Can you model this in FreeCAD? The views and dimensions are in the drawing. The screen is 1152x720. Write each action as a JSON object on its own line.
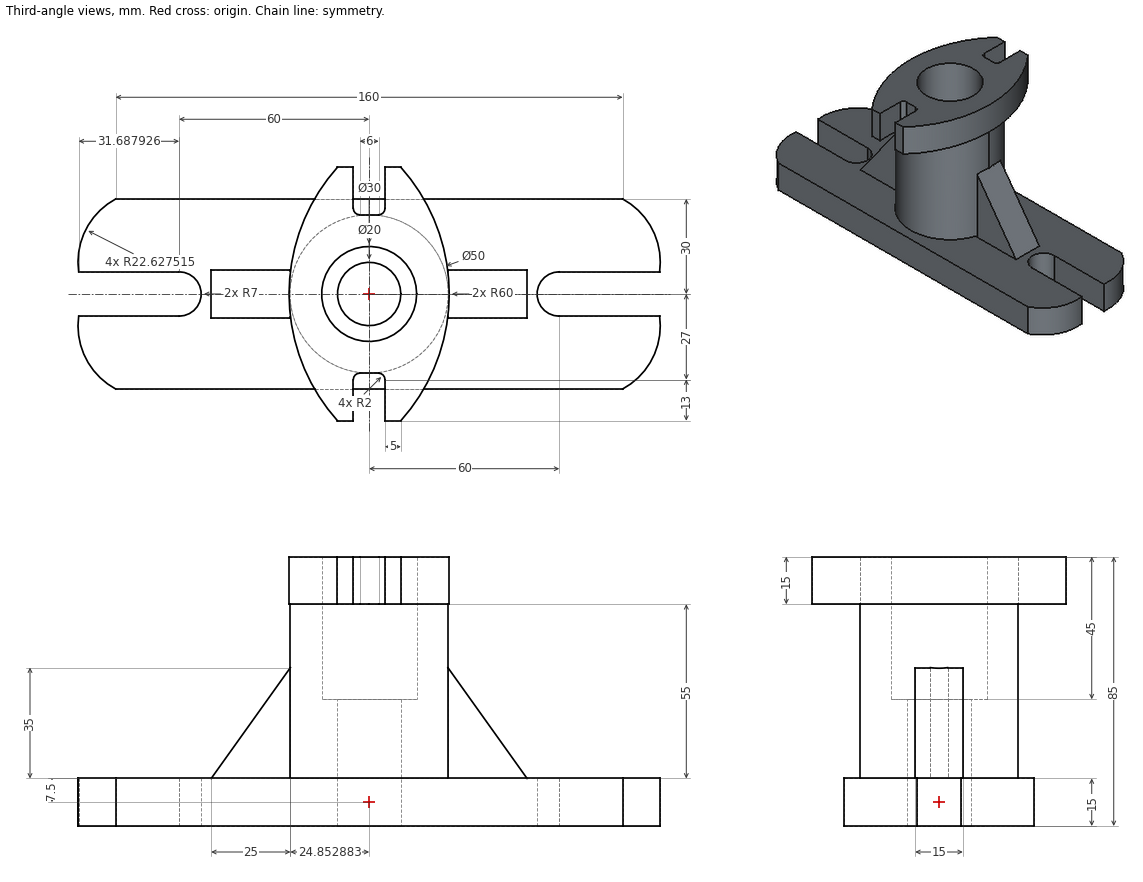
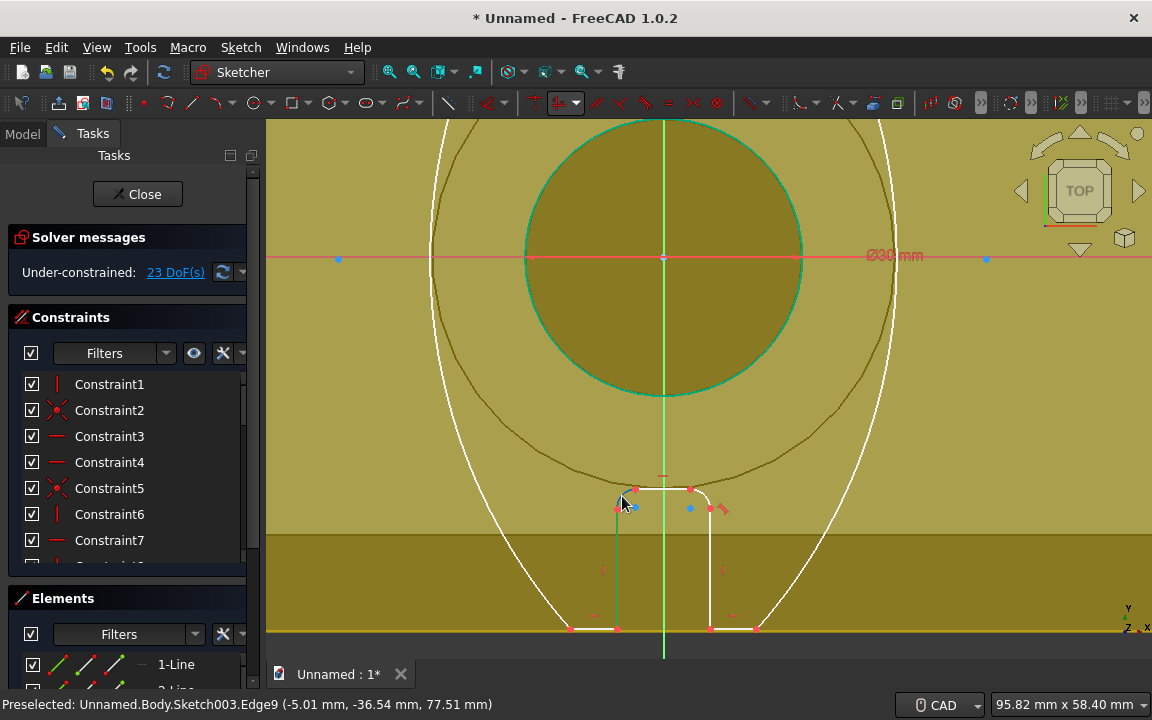
{"action": "left_click", "coordinate": [622, 495]}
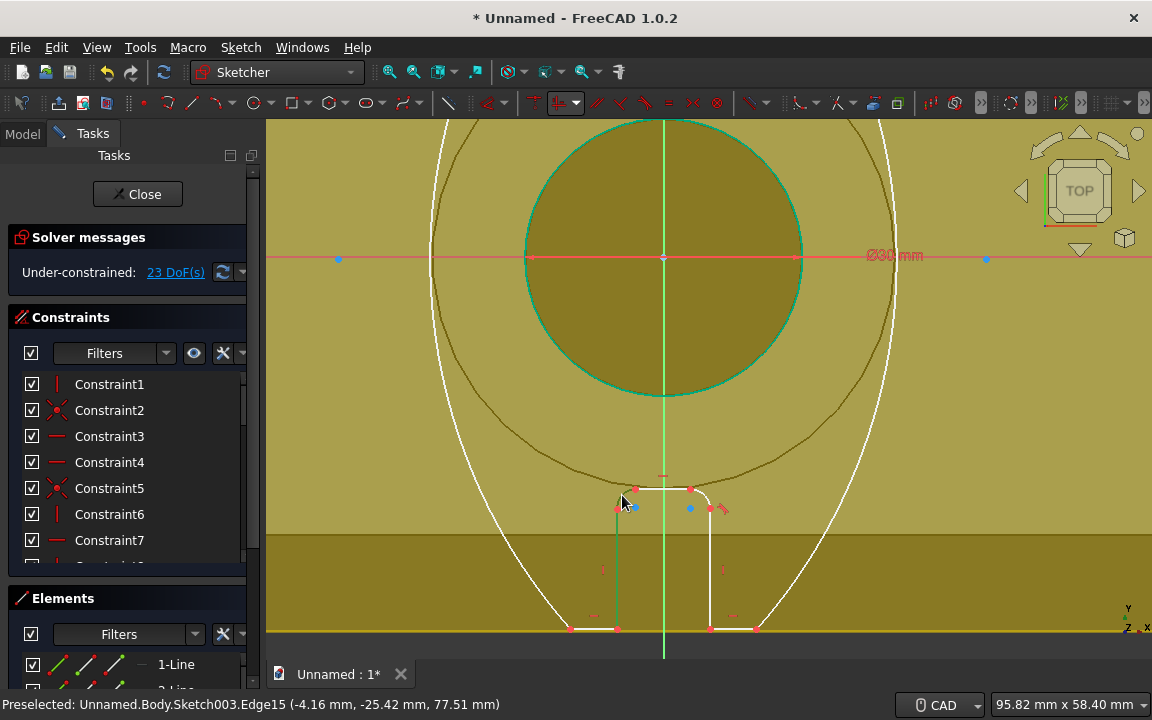
{"action": "key", "text": "t"}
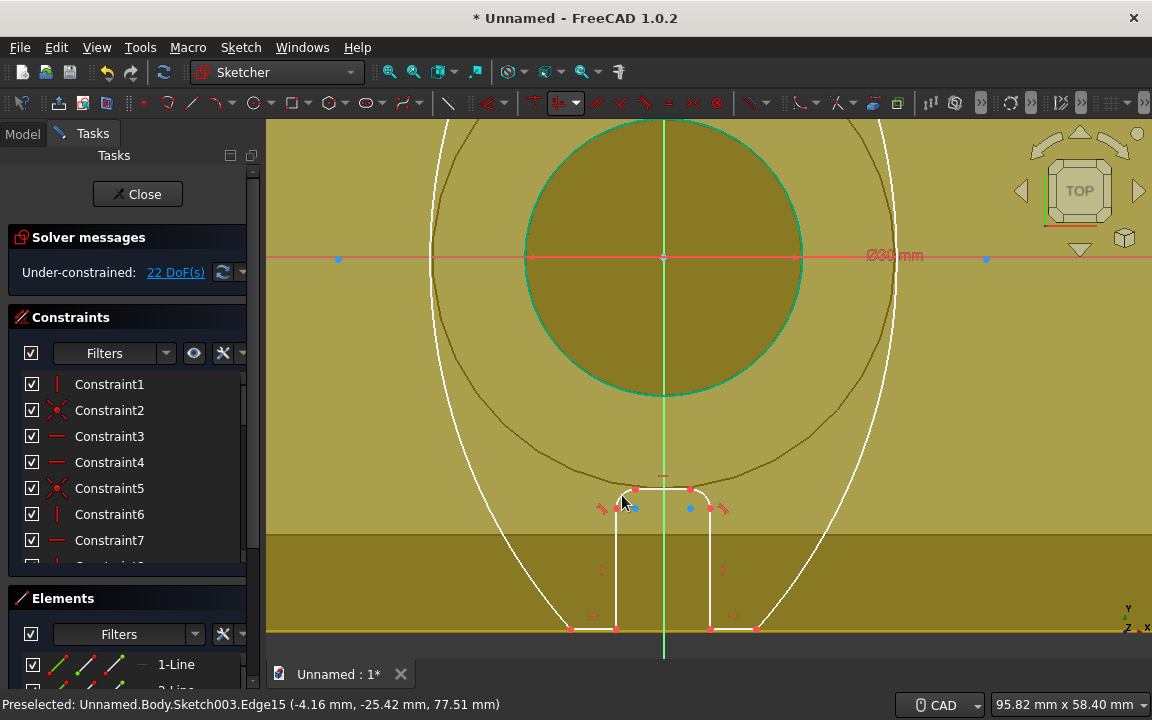
{"action": "left_click", "coordinate": [652, 489]}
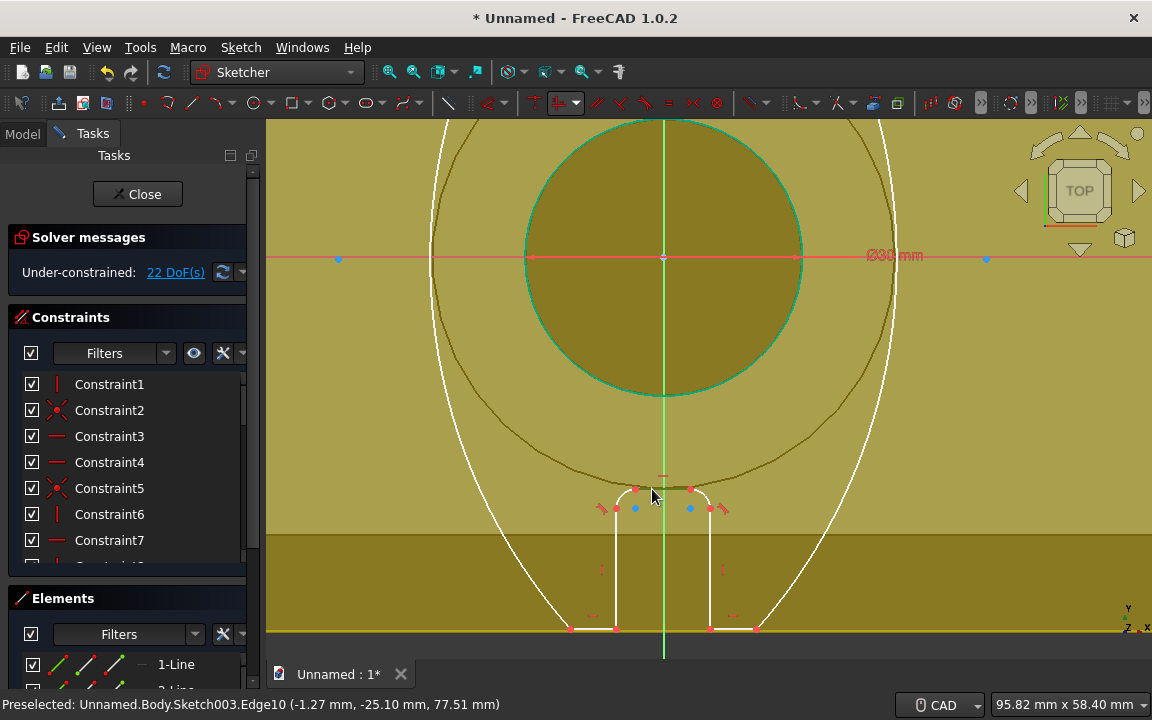
{"action": "scroll", "coordinate": [627, 492], "scroll_direction": "up", "scroll_amount": 3}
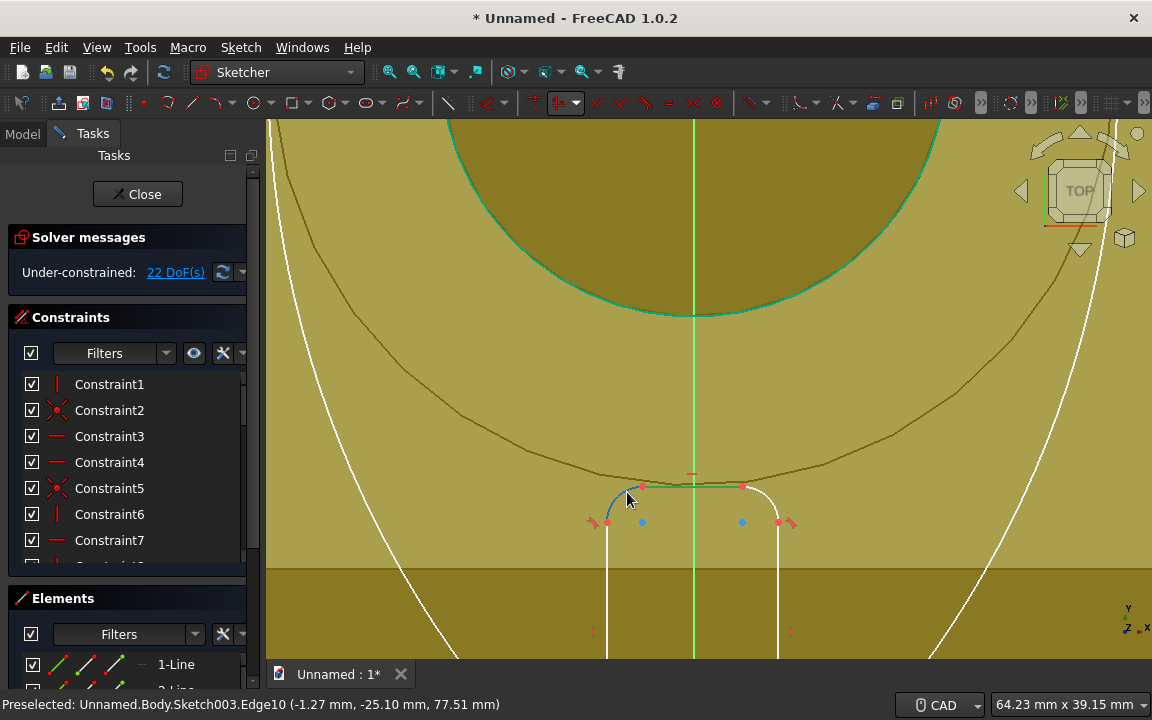
{"action": "left_click", "coordinate": [626, 491]}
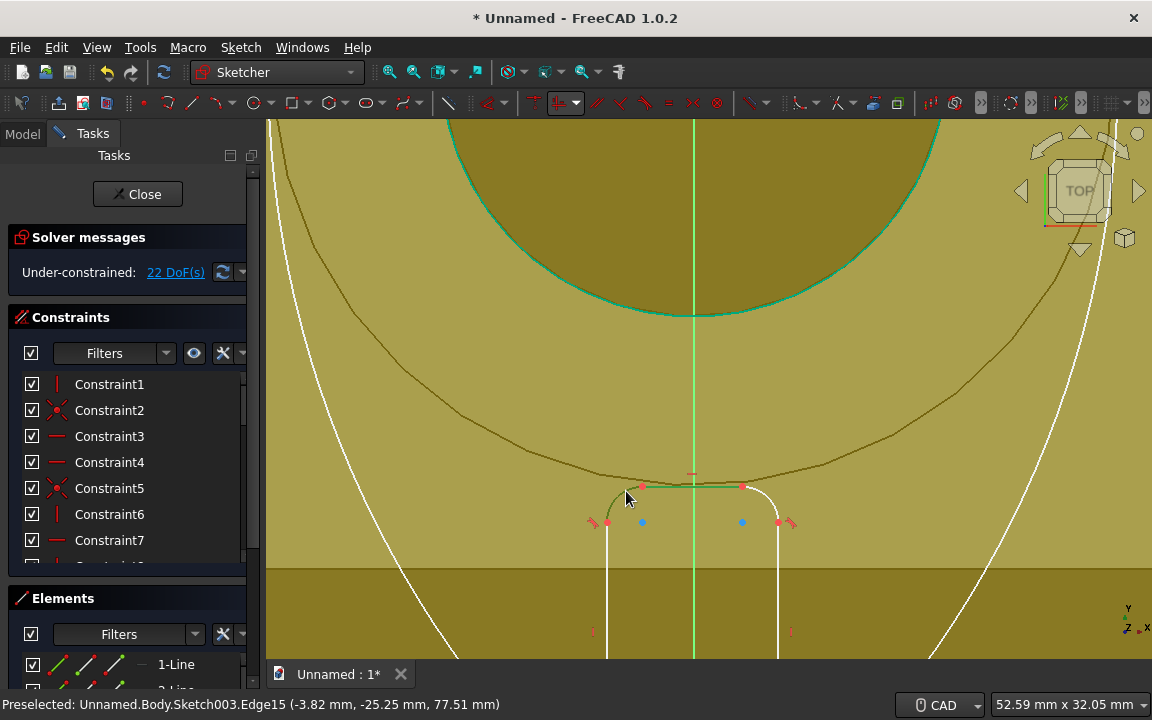
{"action": "left_click", "coordinate": [646, 104]}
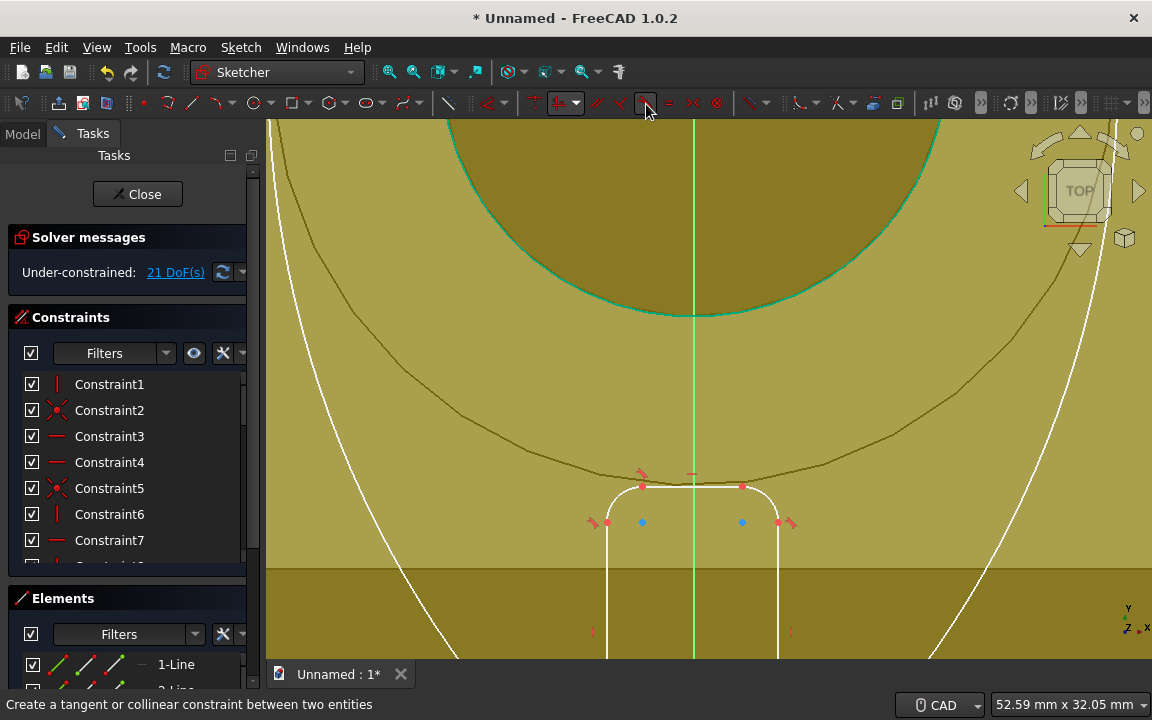
{"action": "left_click", "coordinate": [673, 487]}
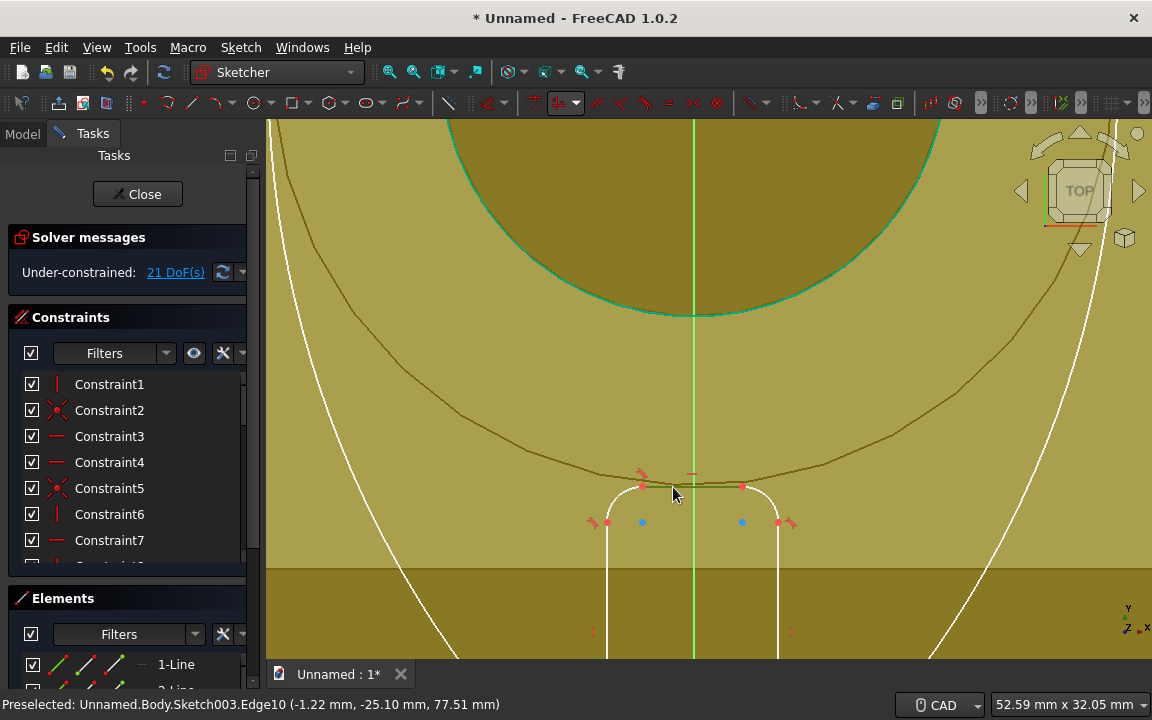
{"action": "left_click", "coordinate": [774, 506]}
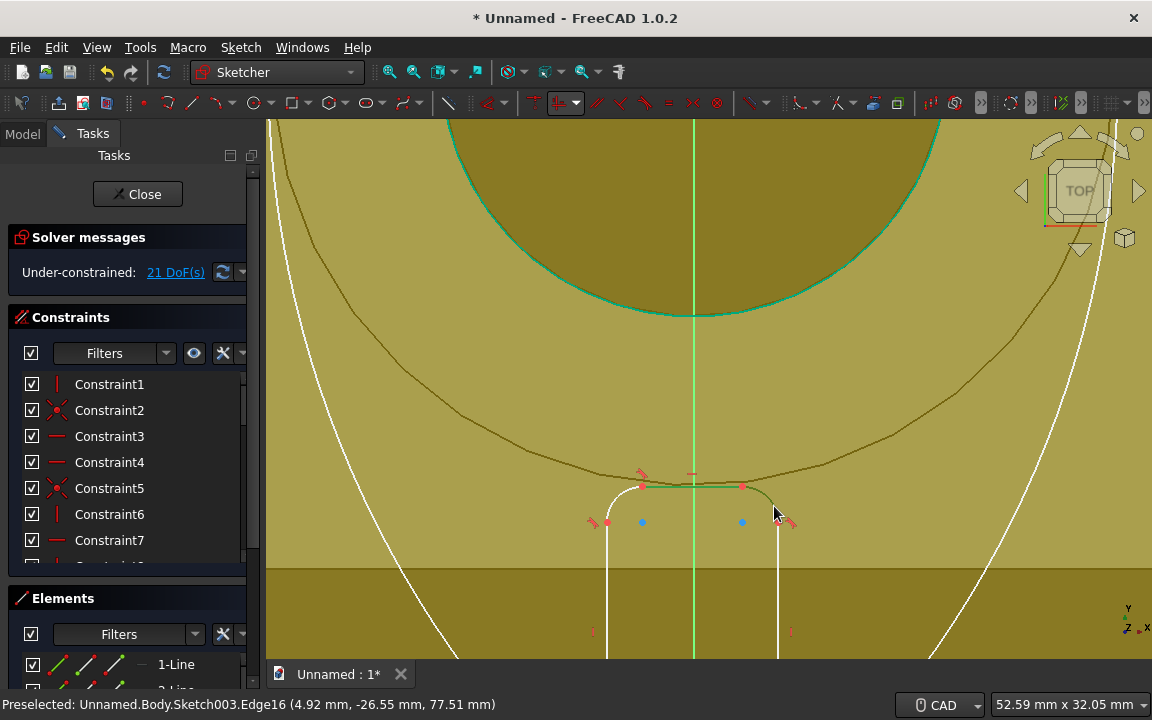
{"action": "key", "text": "t"}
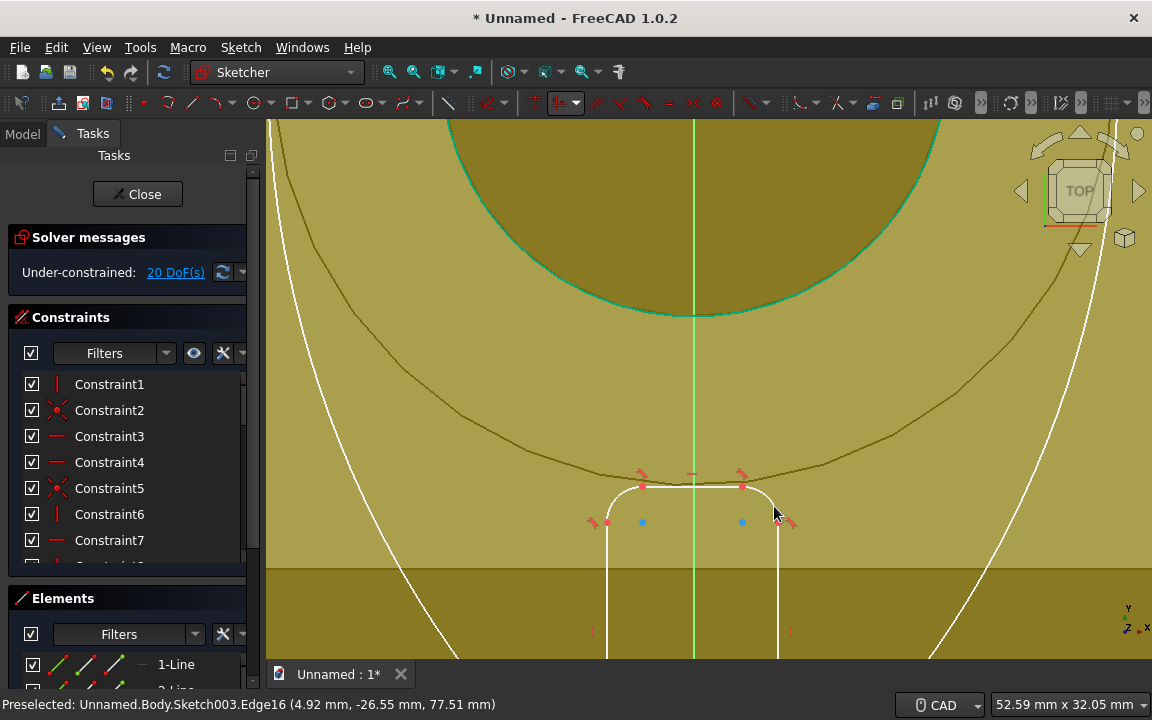
{"action": "scroll", "coordinate": [623, 495], "scroll_direction": "down", "scroll_amount": 7}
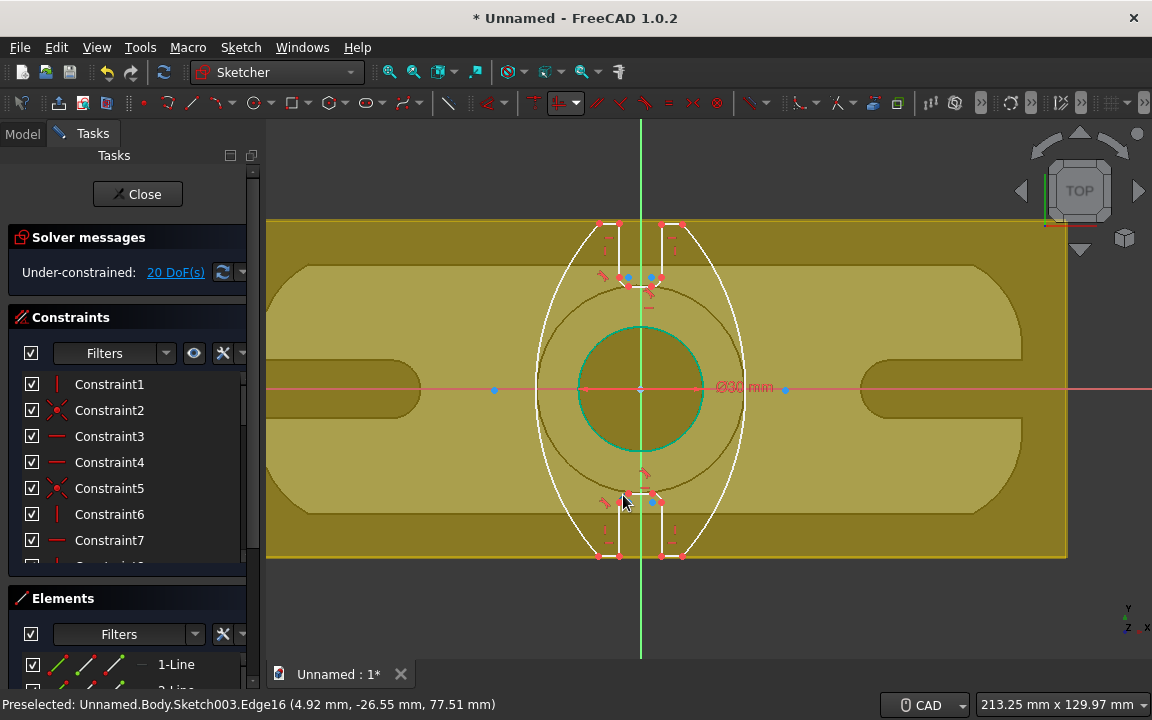
{"action": "scroll", "coordinate": [656, 286], "scroll_direction": "up", "scroll_amount": 6}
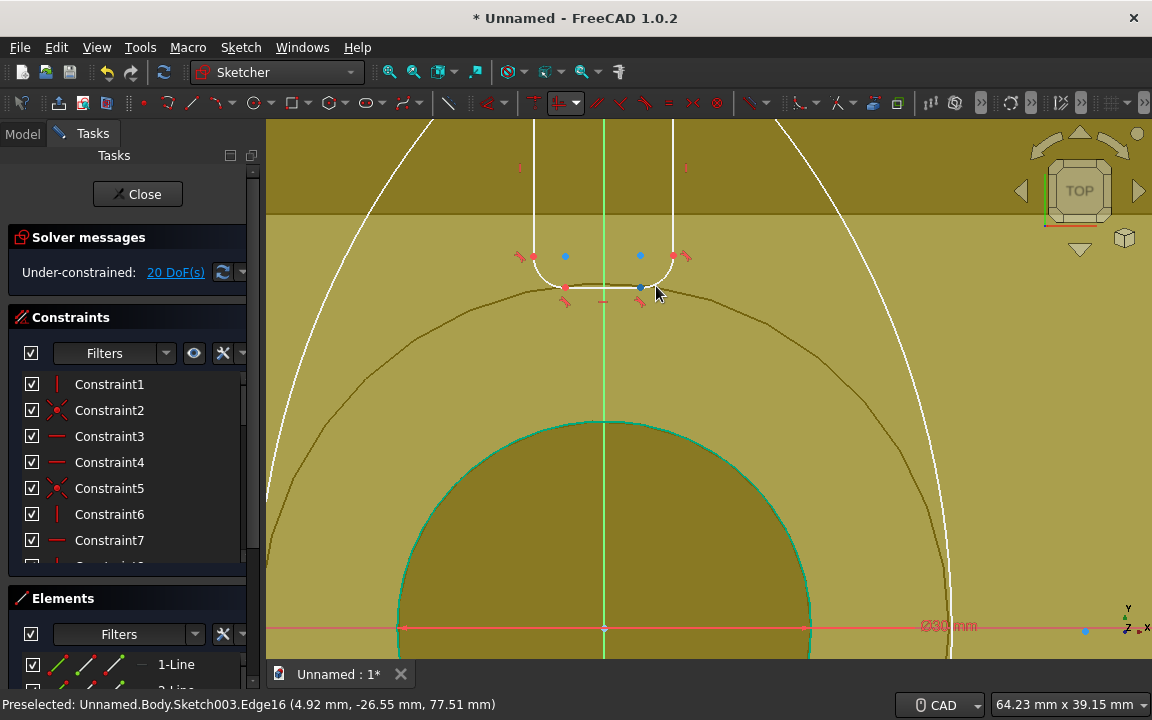
{"action": "left_click", "coordinate": [656, 284]}